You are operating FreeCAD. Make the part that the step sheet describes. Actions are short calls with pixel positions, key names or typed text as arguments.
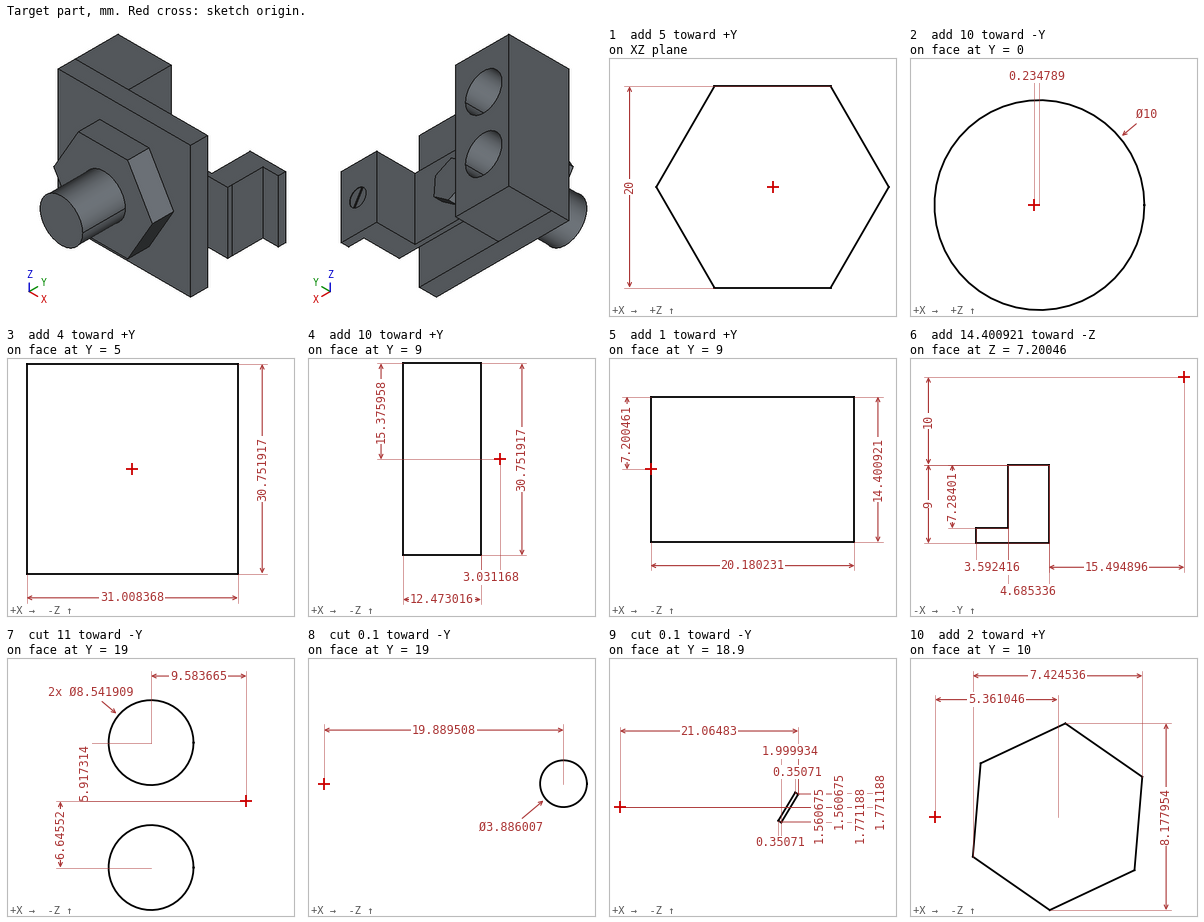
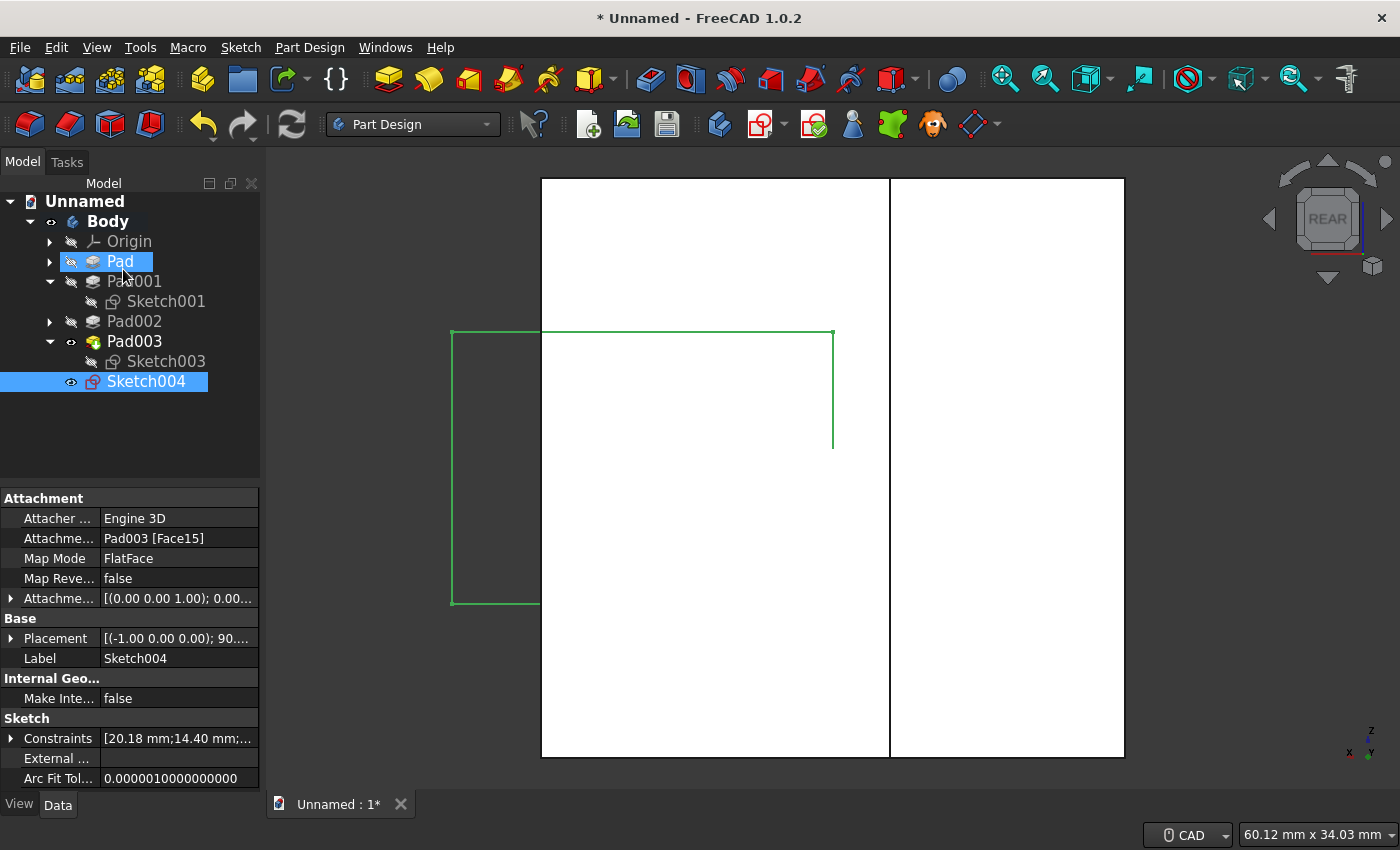
click(390, 80)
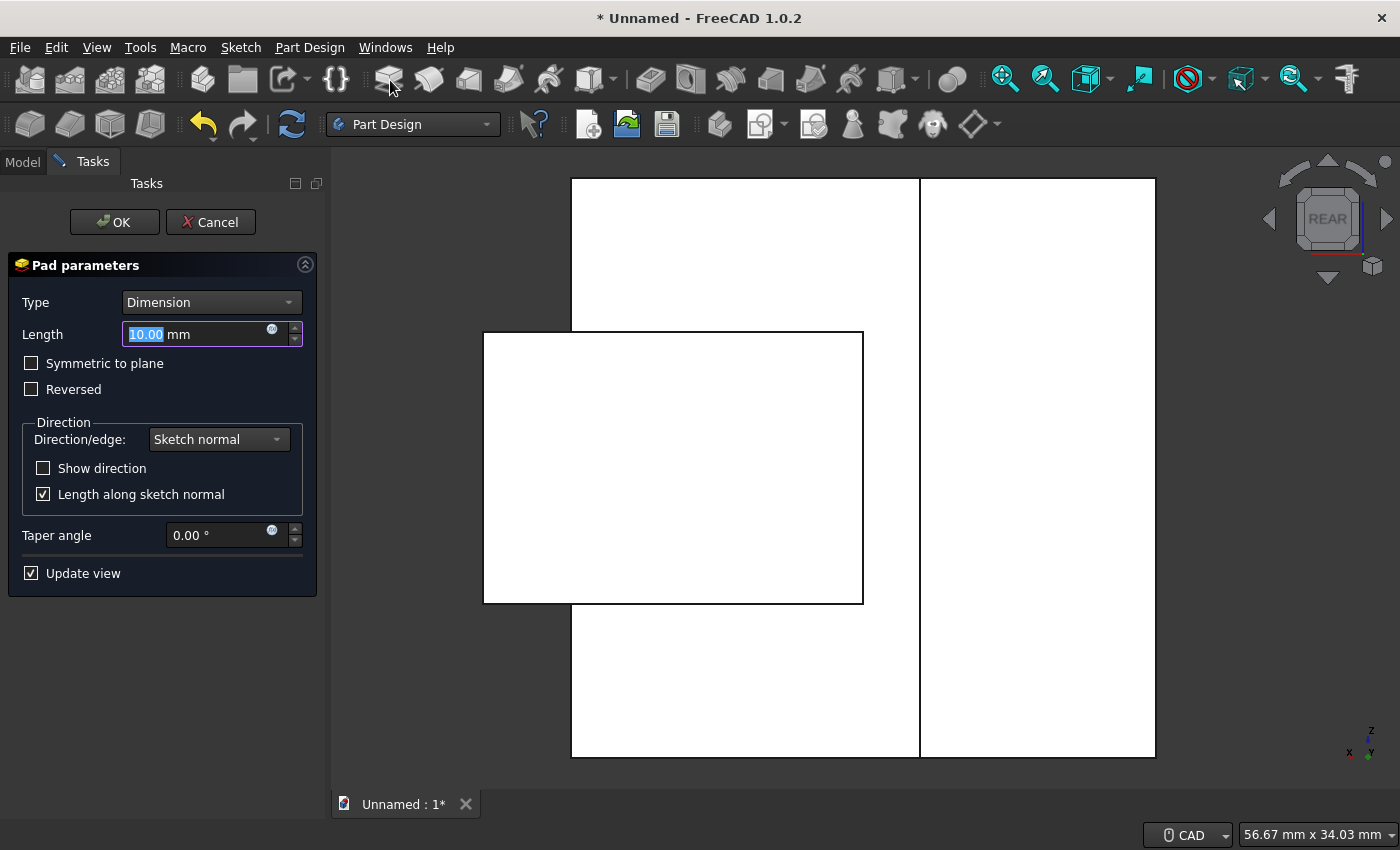
text(1)
key(Tab)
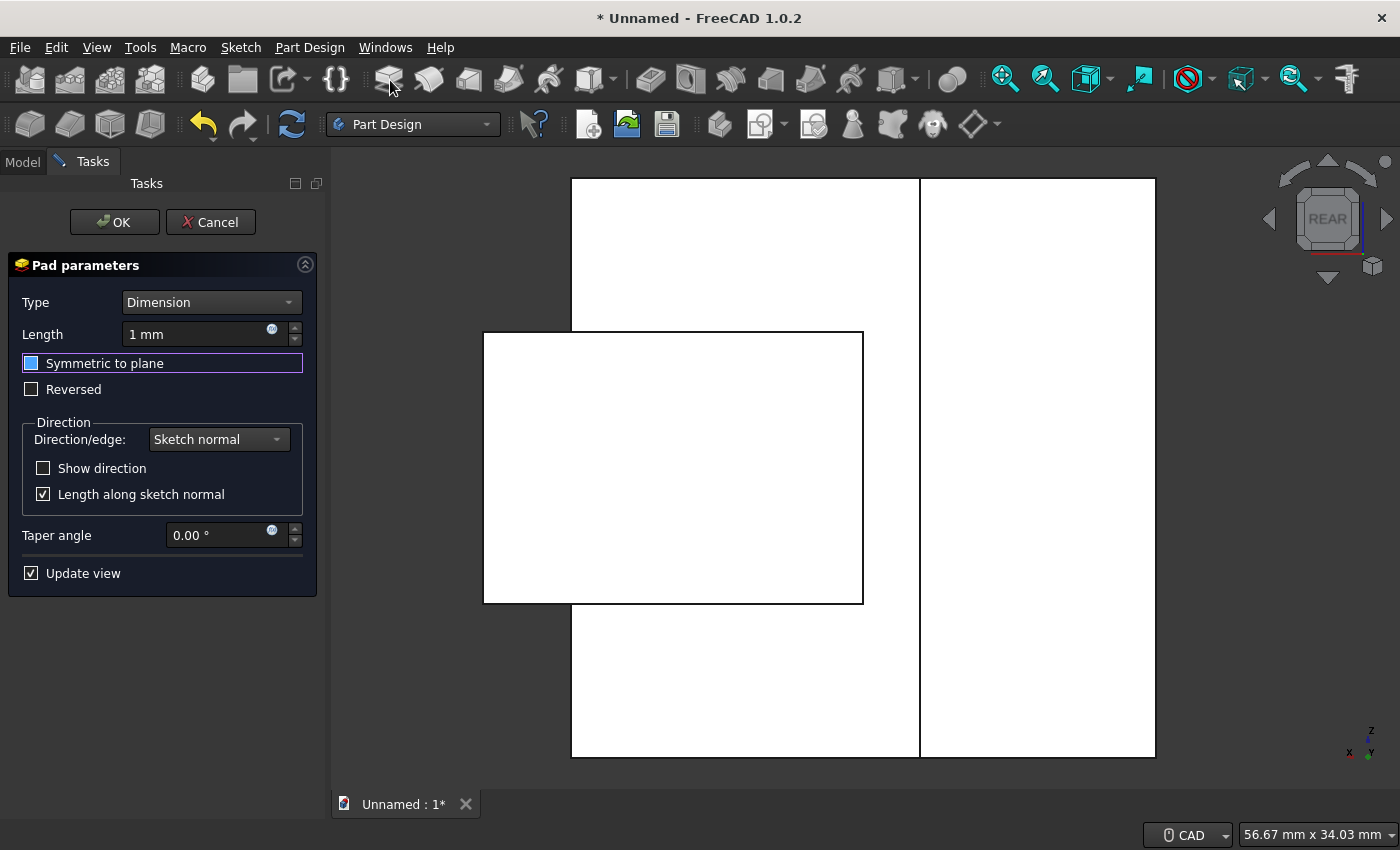
click(115, 222)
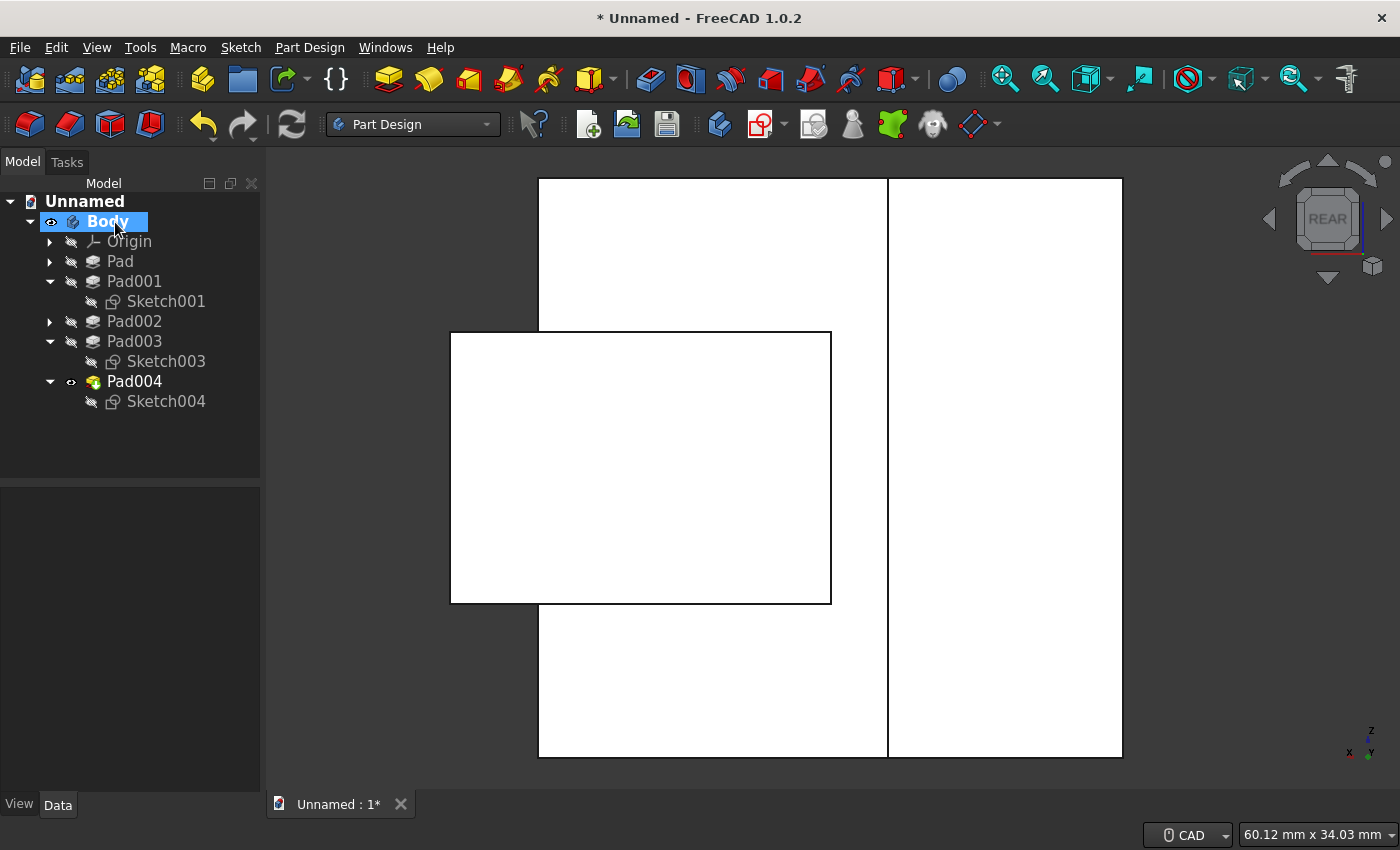
key(0)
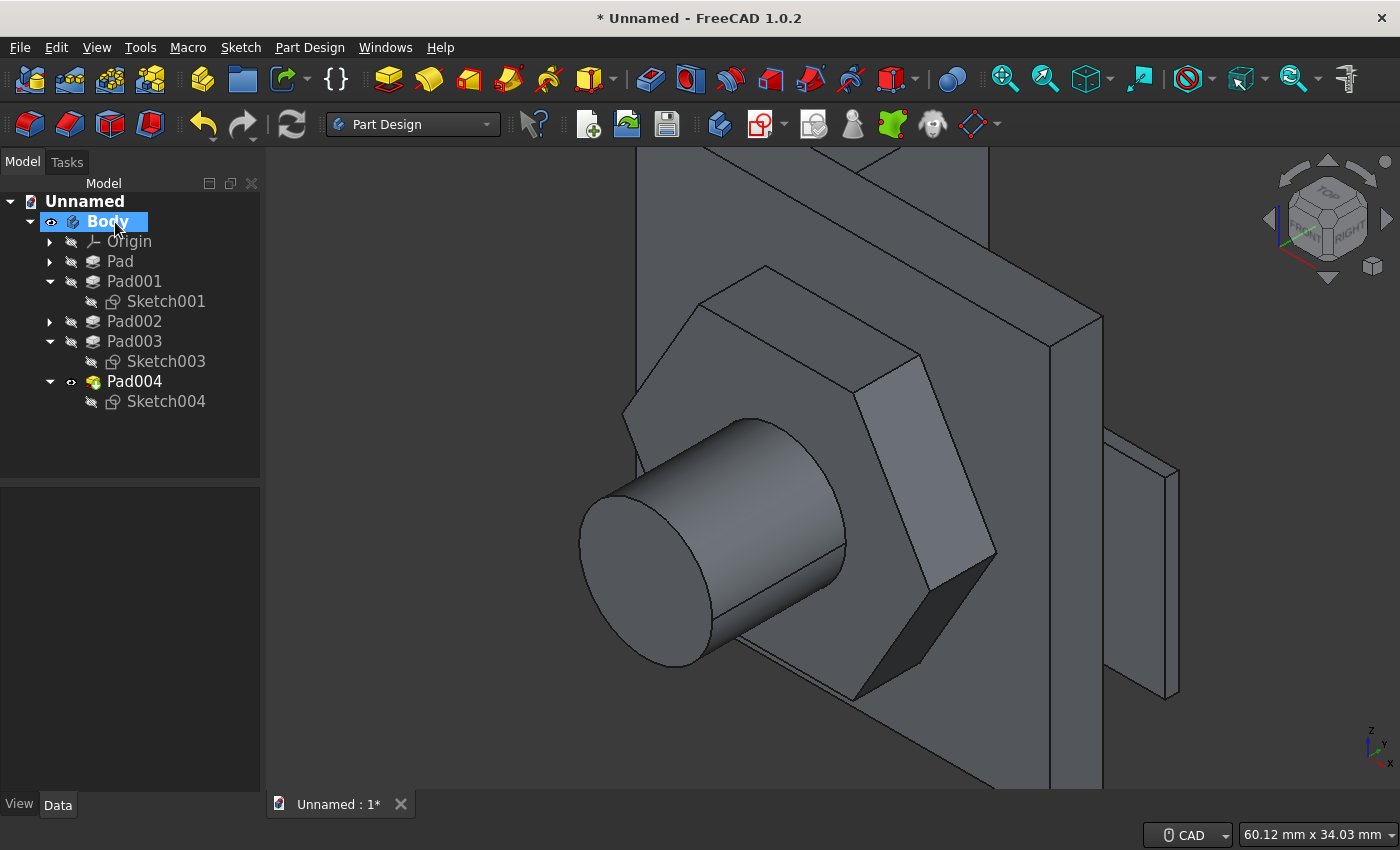
click(1006, 80)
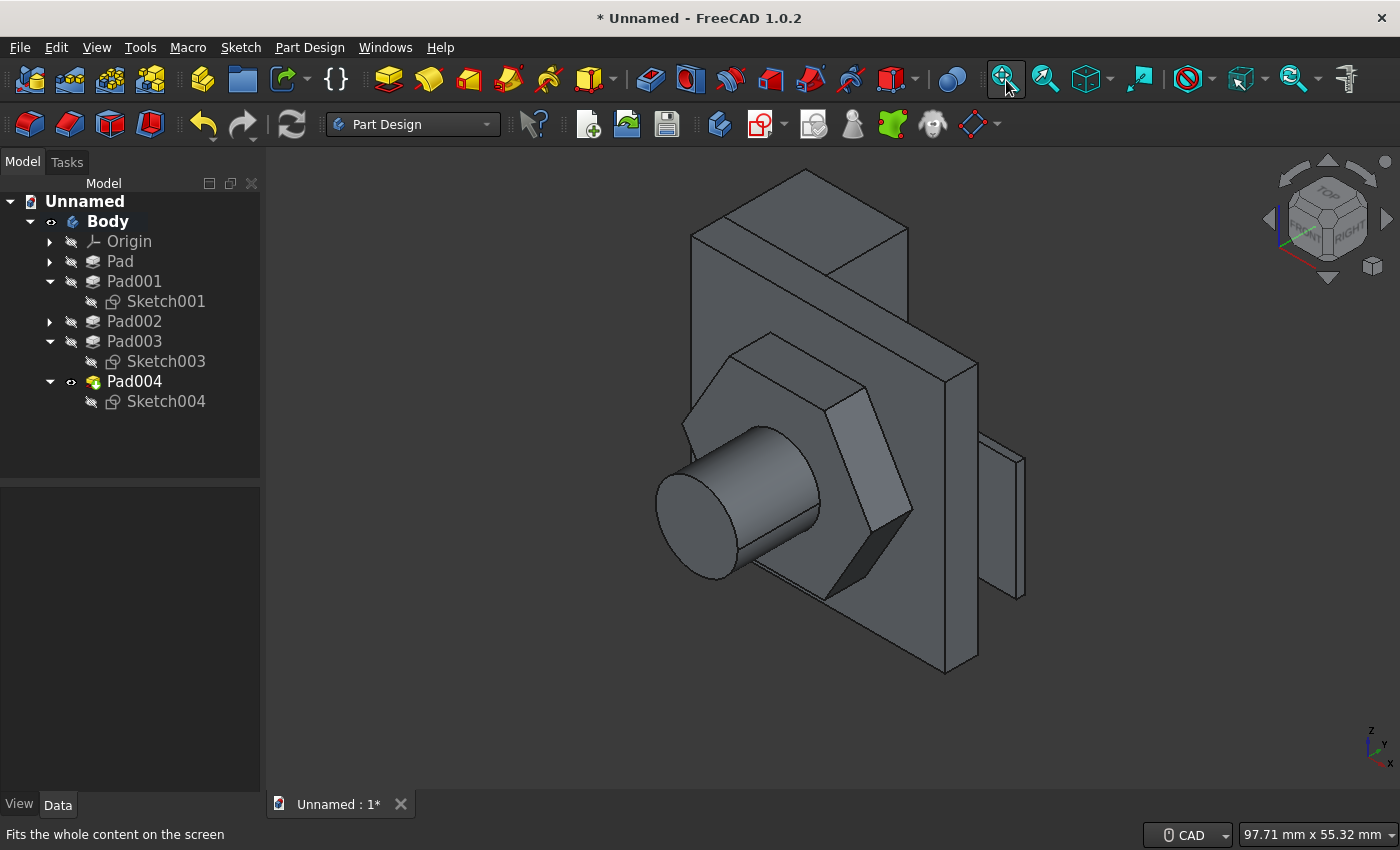
scroll(1009, 453, up, 4)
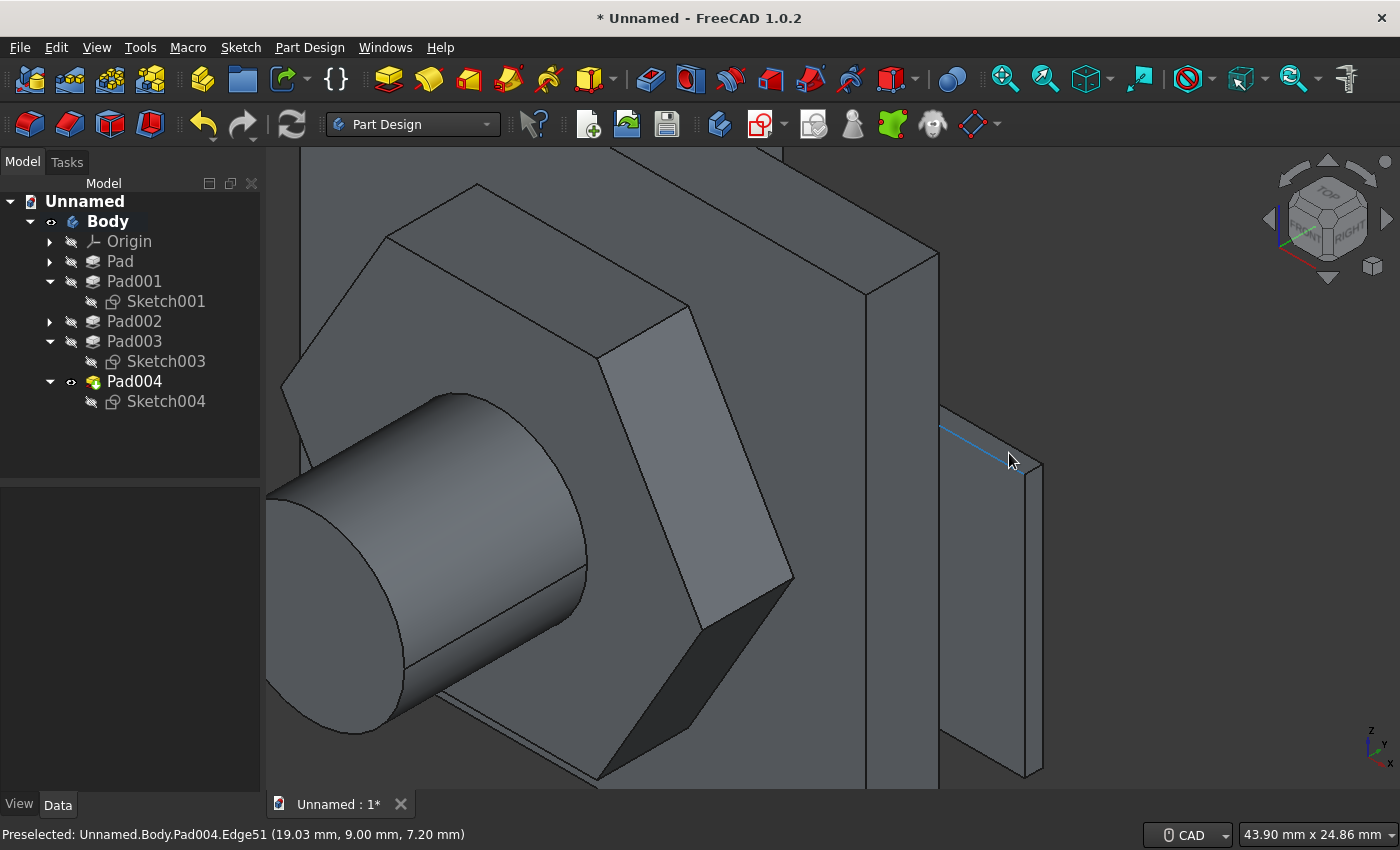
click(1010, 452)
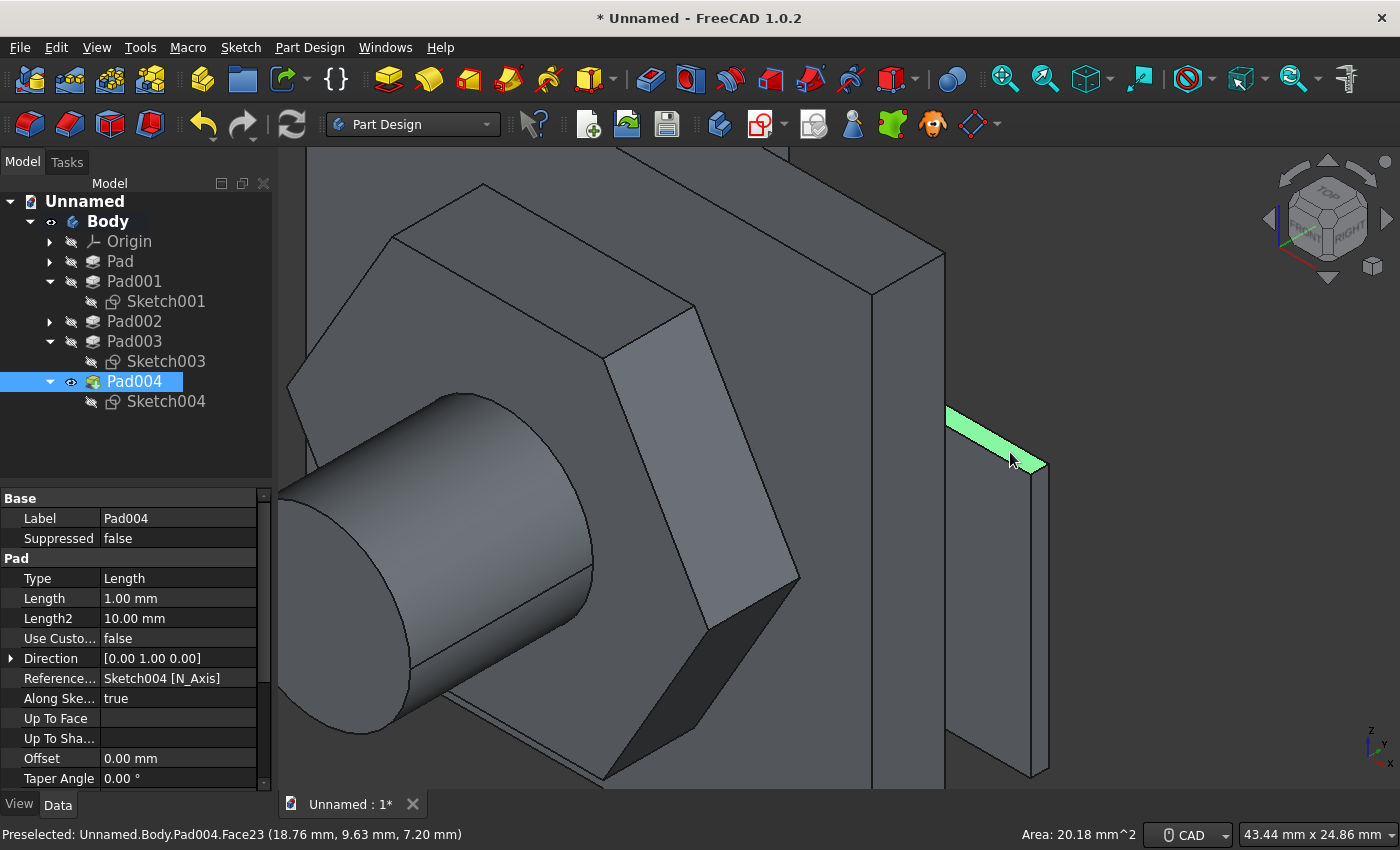
click(760, 124)